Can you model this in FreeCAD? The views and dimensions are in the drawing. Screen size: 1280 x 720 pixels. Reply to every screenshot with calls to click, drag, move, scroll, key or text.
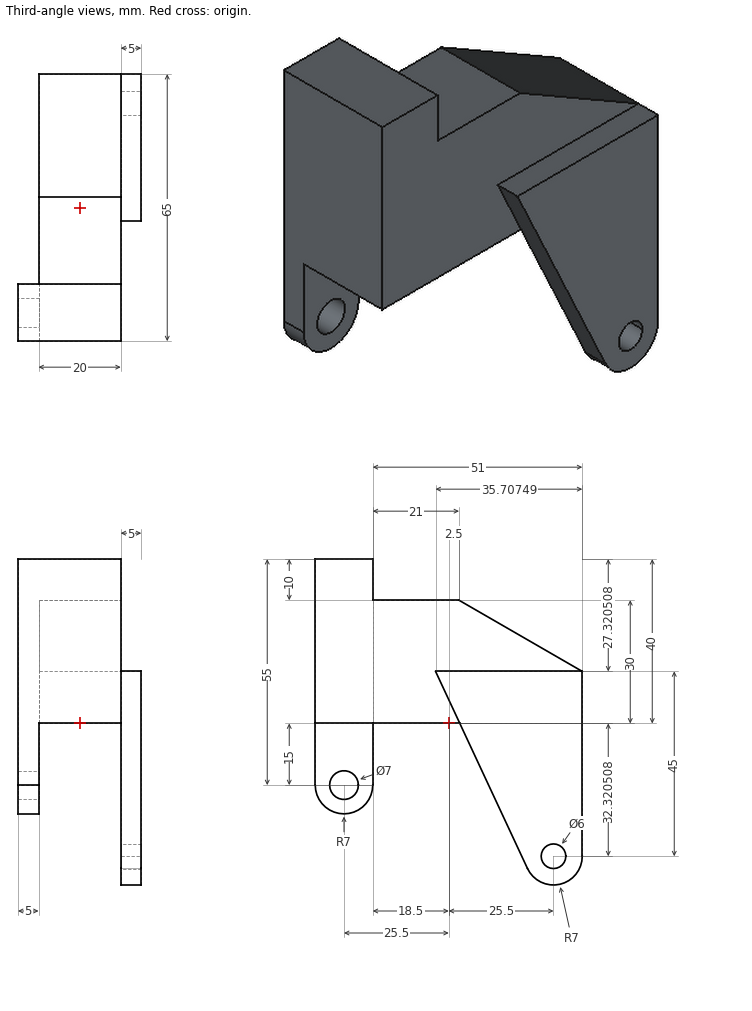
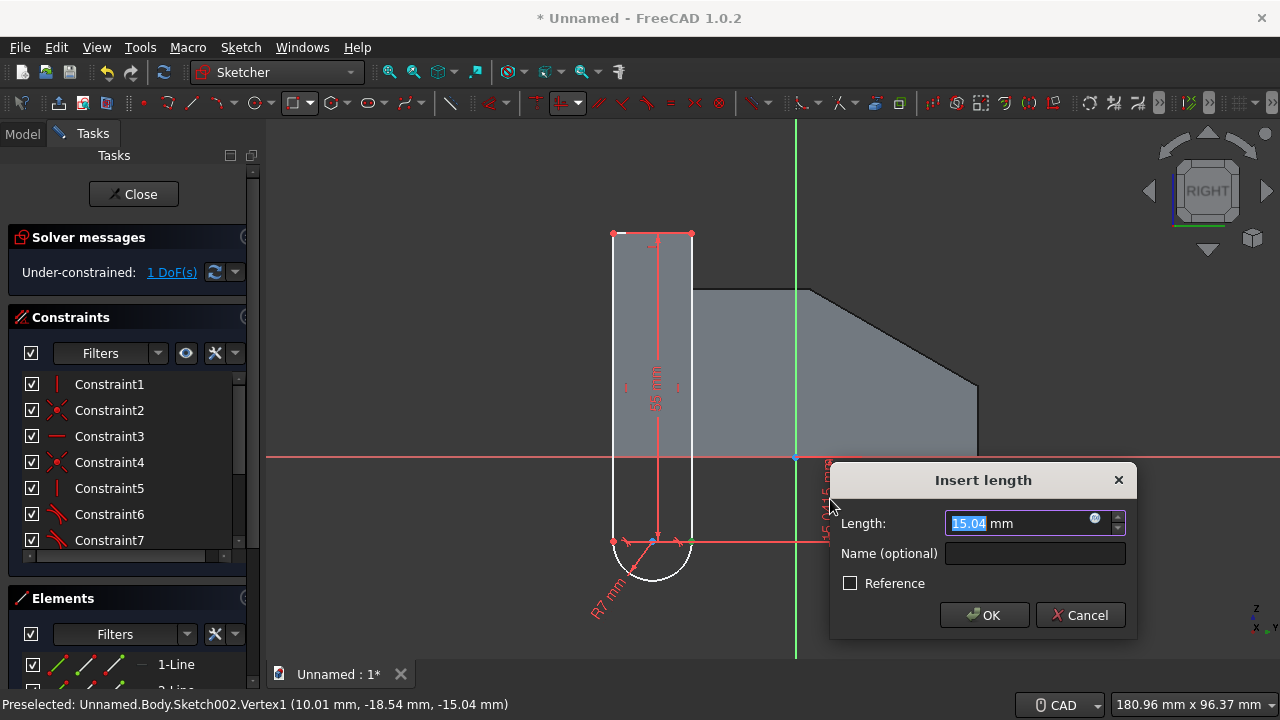
text(15)
key(Return)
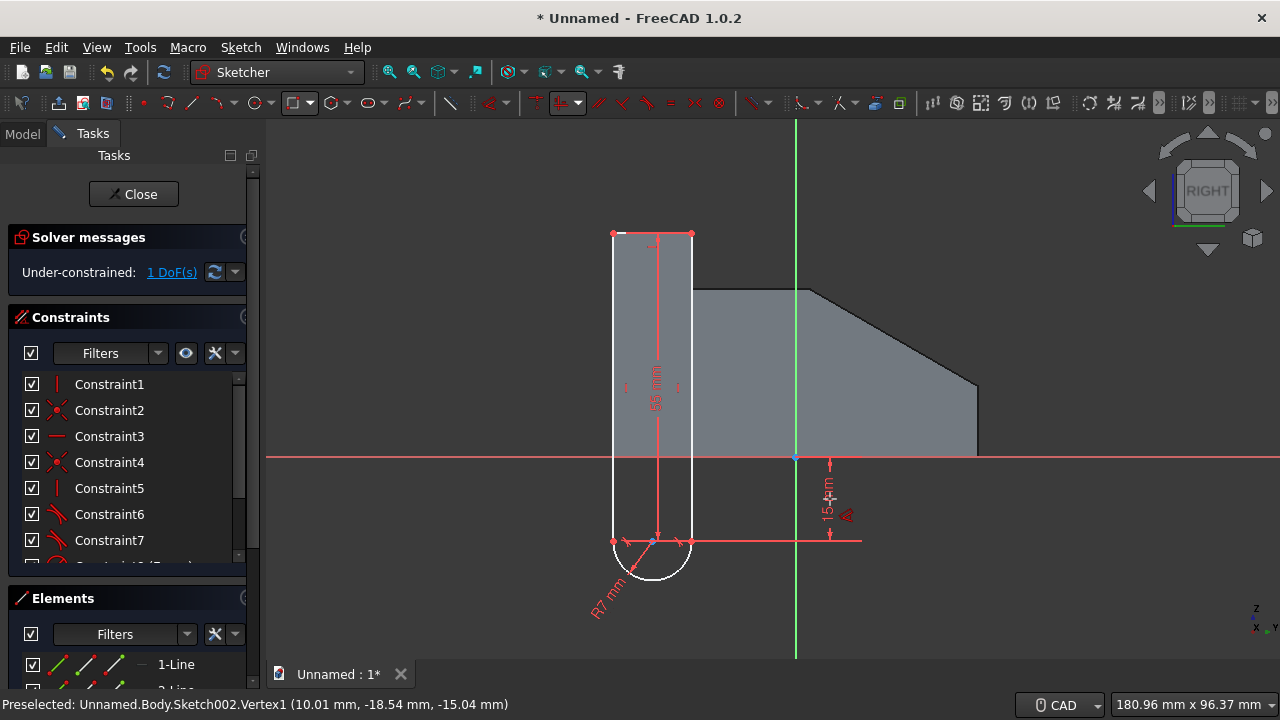
click(692, 541)
click(744, 575)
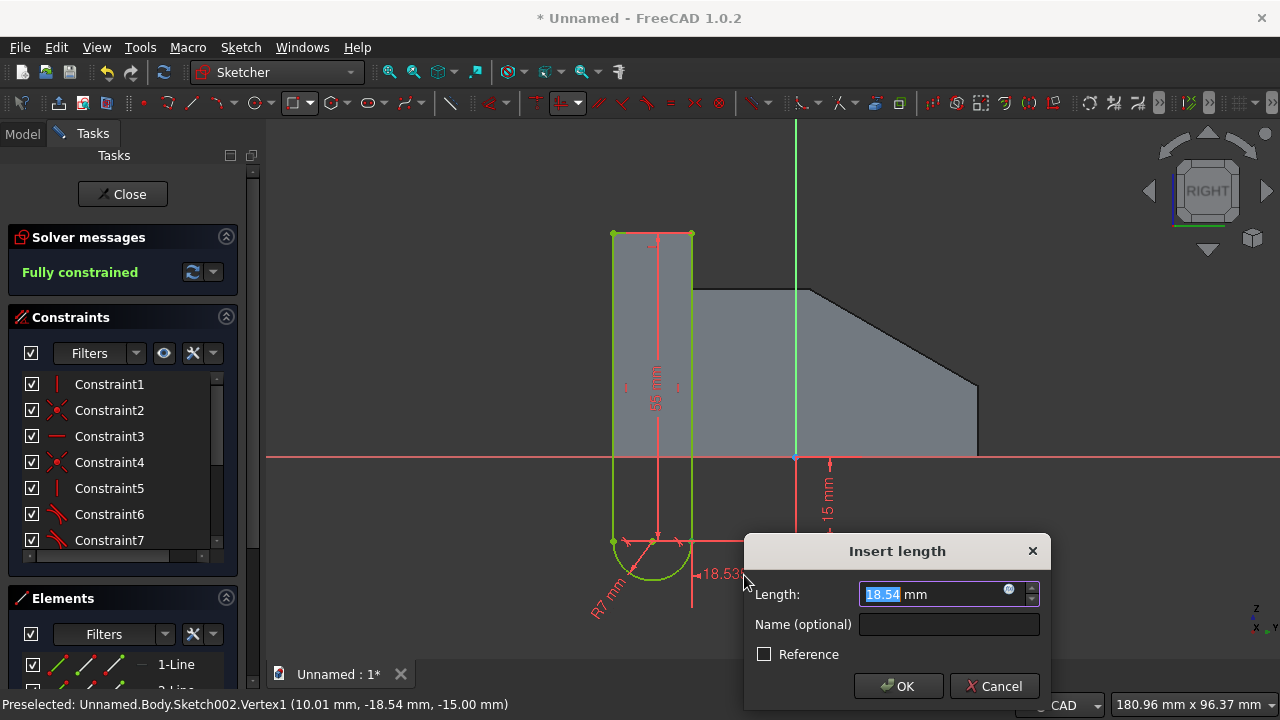
text(18.5)
key(Return)
key(Escape)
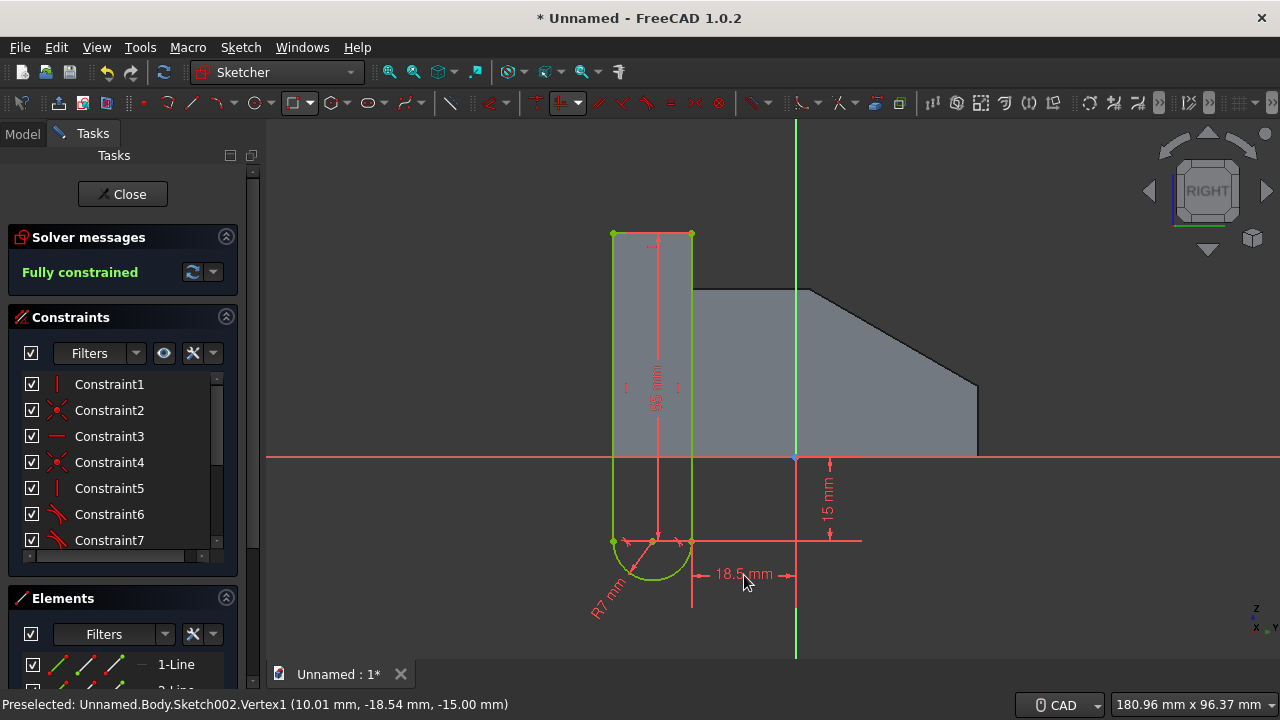
click(123, 194)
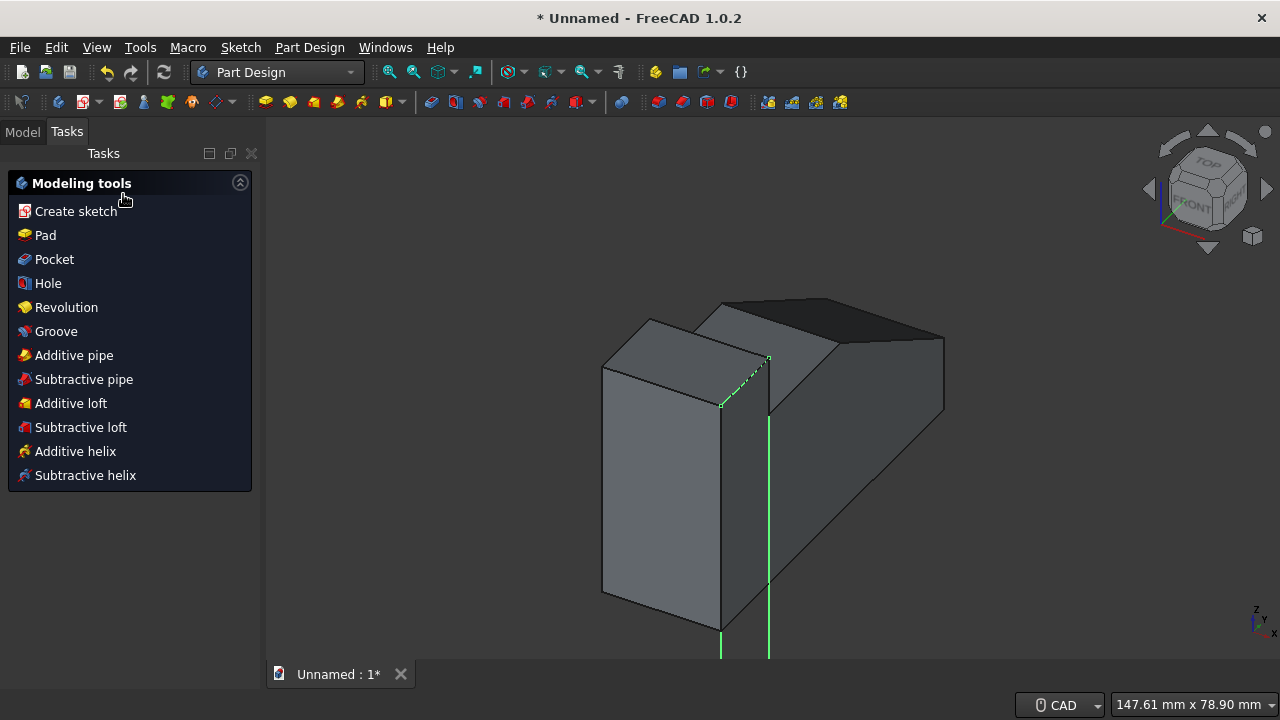
click(266, 102)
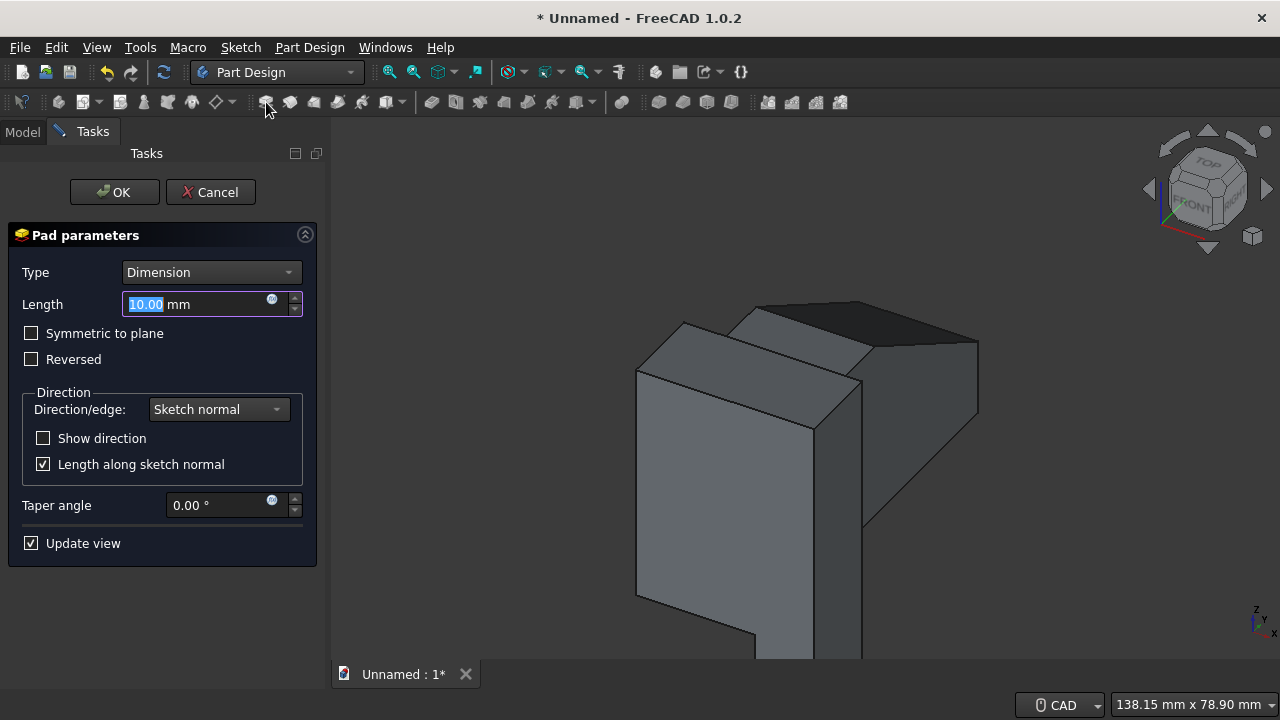
text(5)
key(Tab)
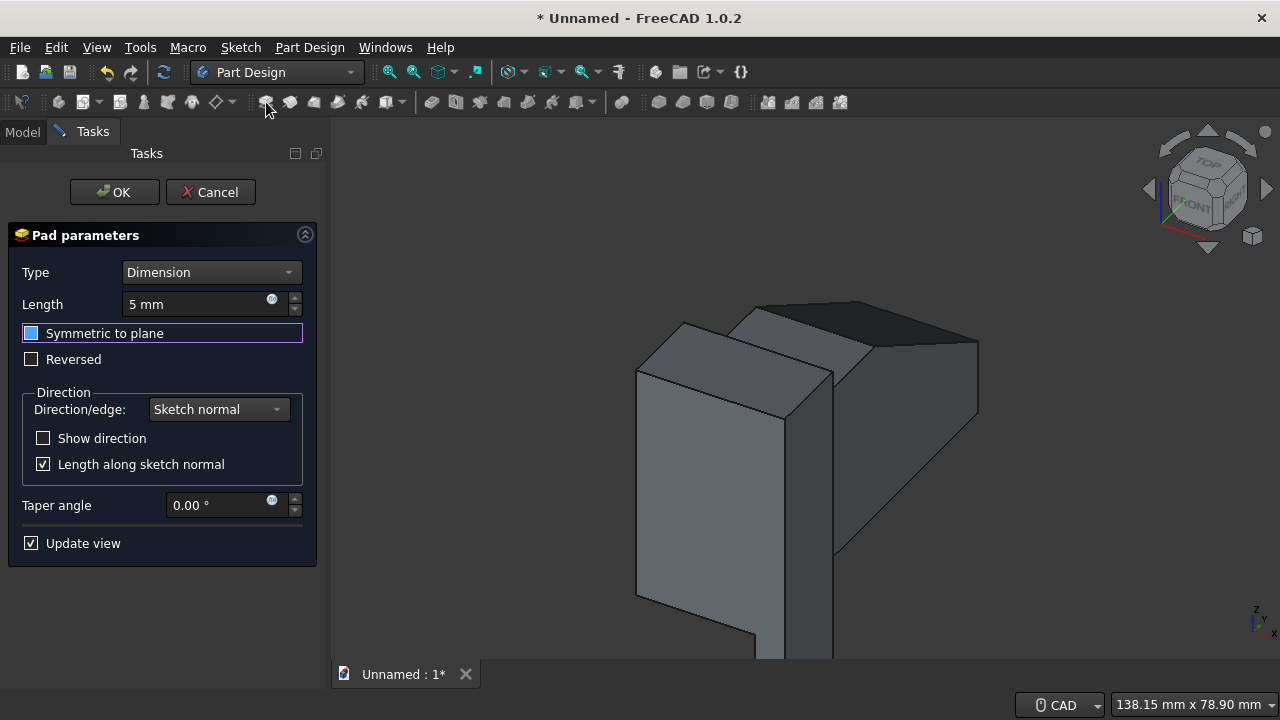
click(115, 192)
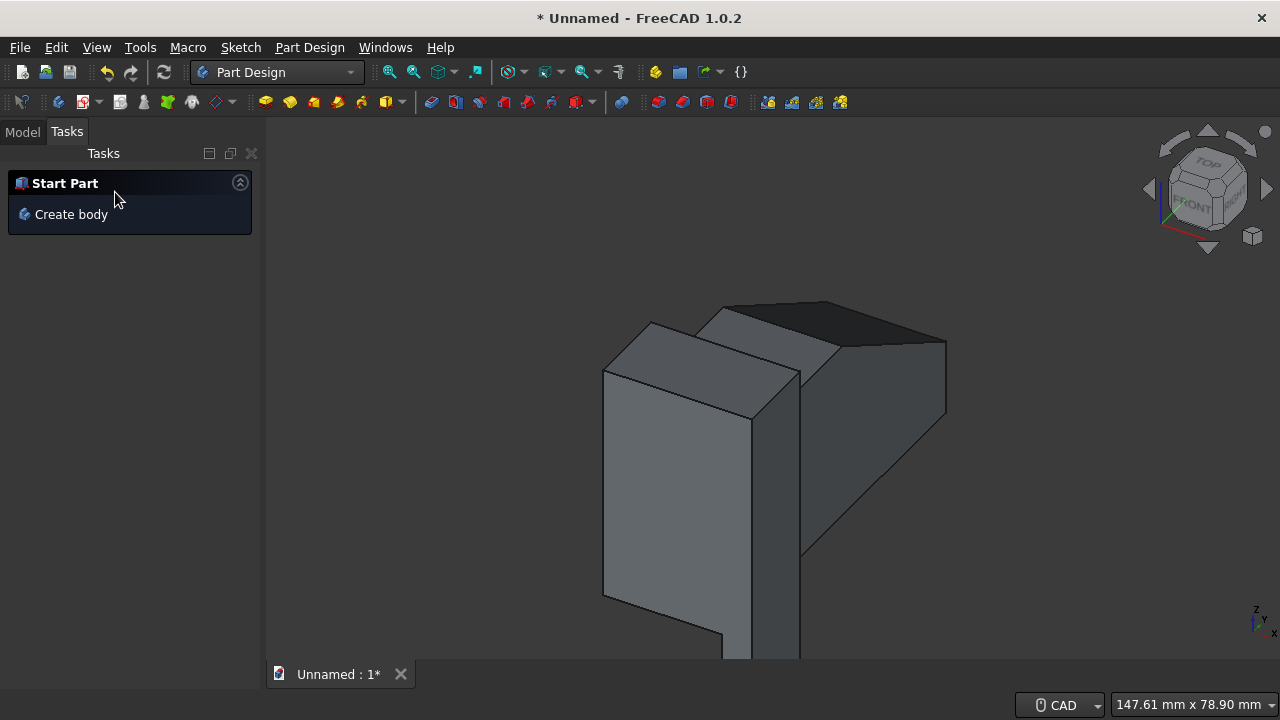
click(390, 72)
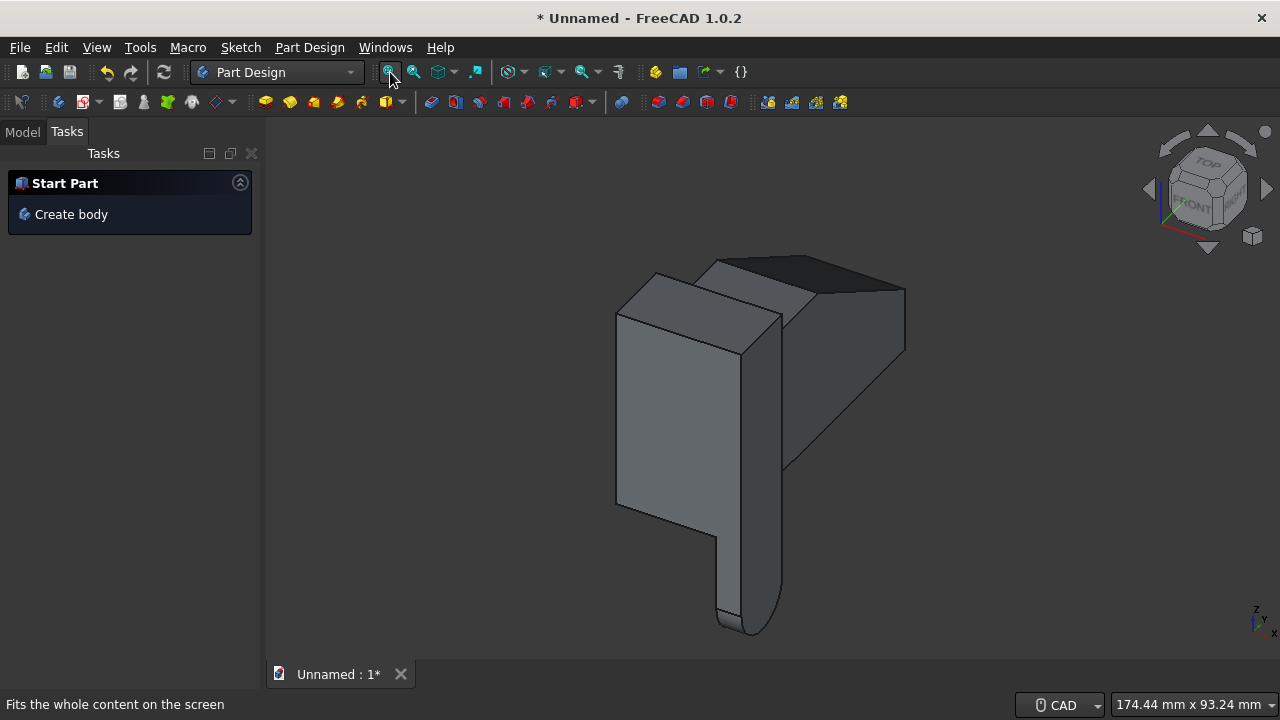
click(23, 131)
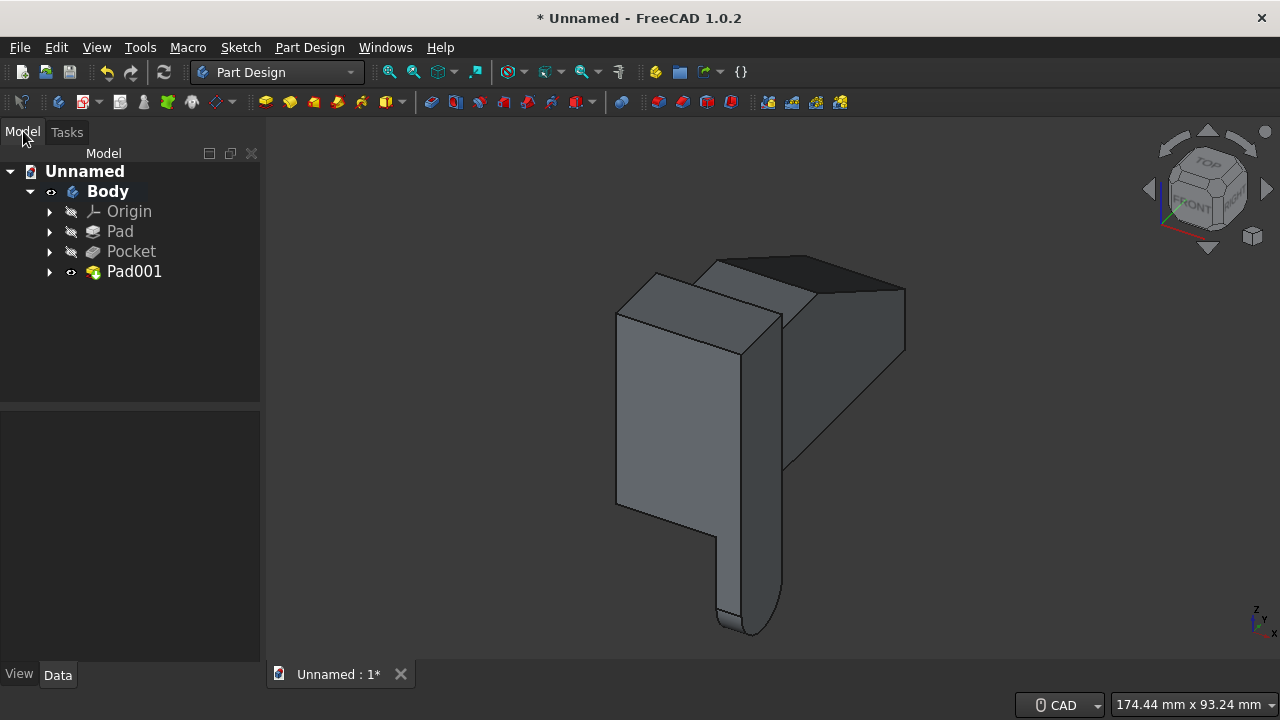
click(116, 272)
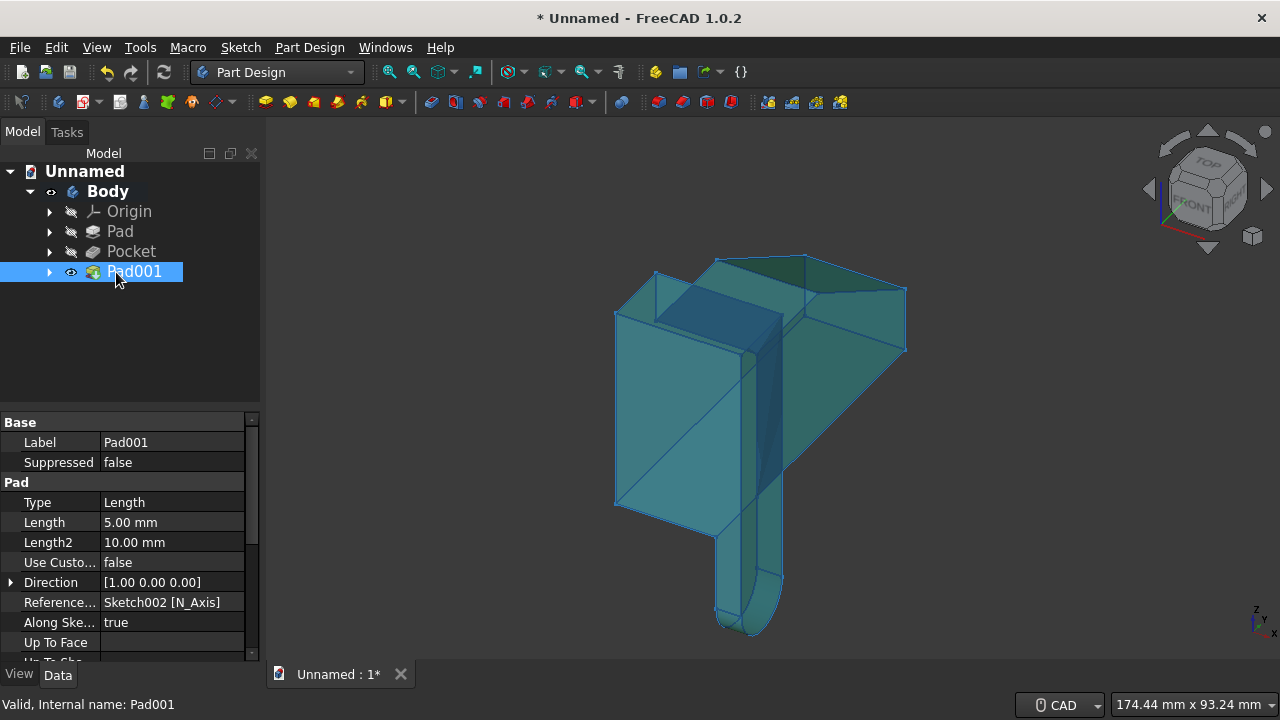
click(768, 102)